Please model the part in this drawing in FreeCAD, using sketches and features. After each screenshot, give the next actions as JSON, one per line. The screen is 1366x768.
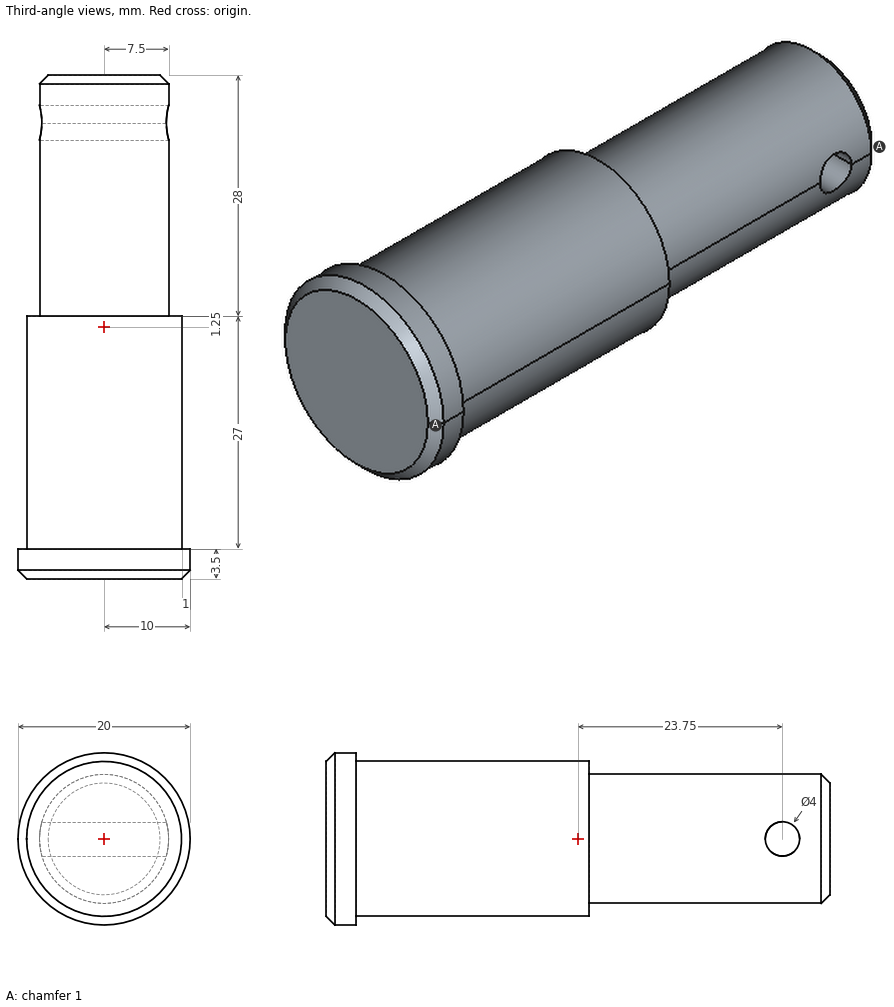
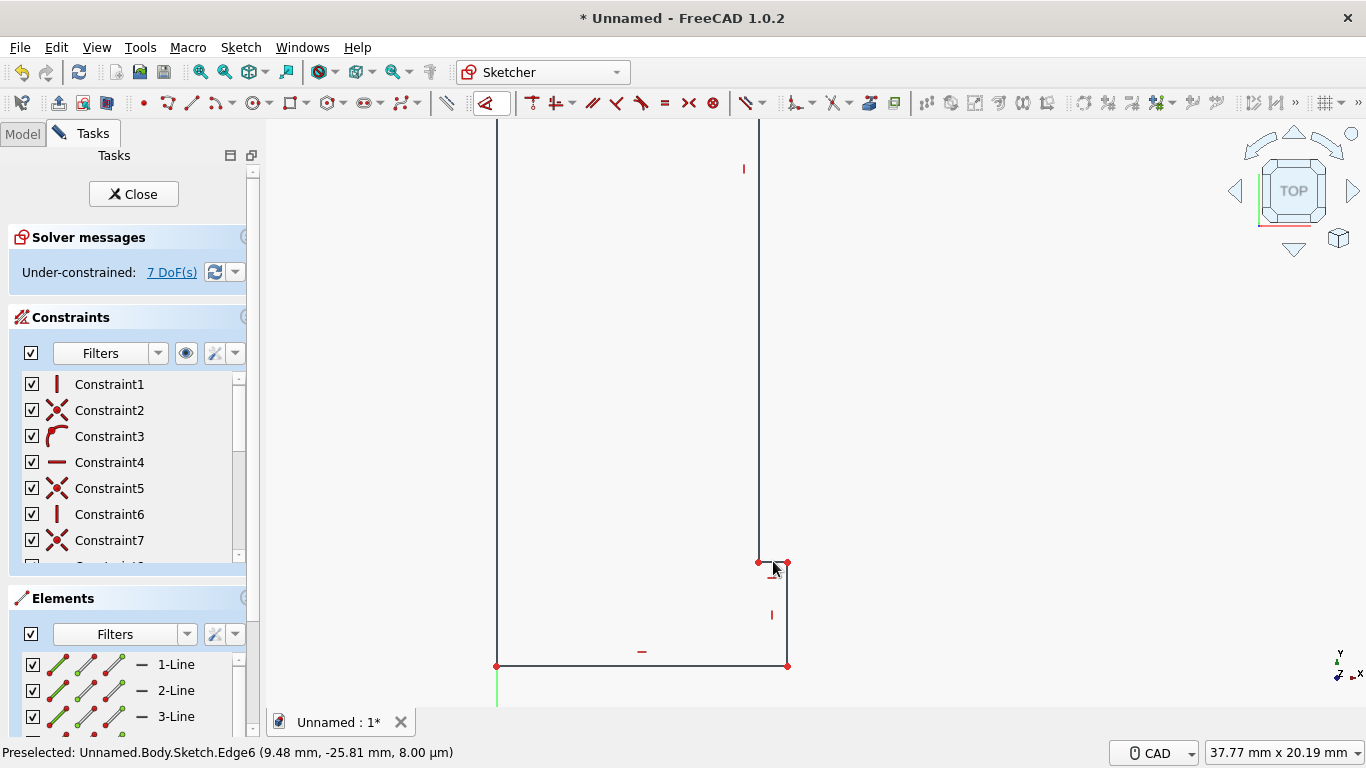
{"action": "left_click", "coordinate": [486, 104]}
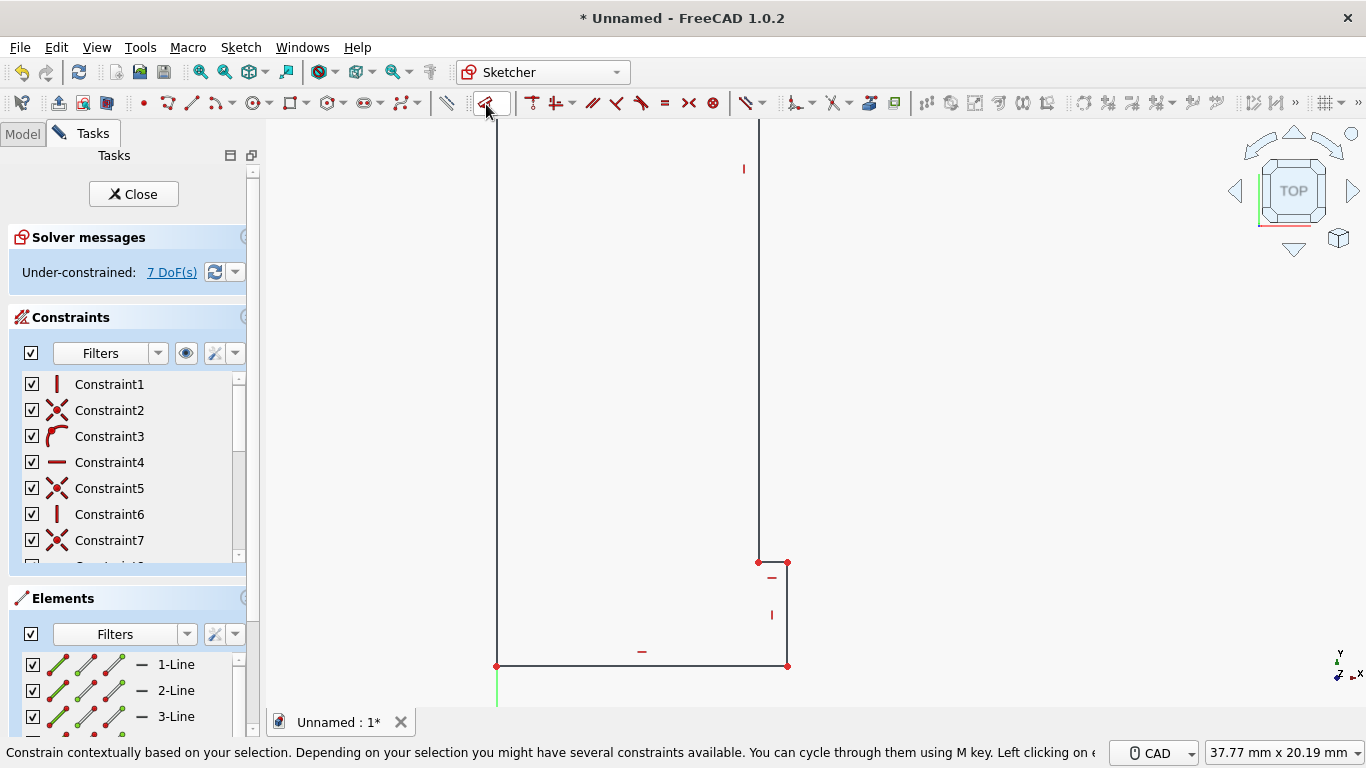
{"action": "scroll", "coordinate": [776, 562], "scroll_direction": "up", "scroll_amount": 2}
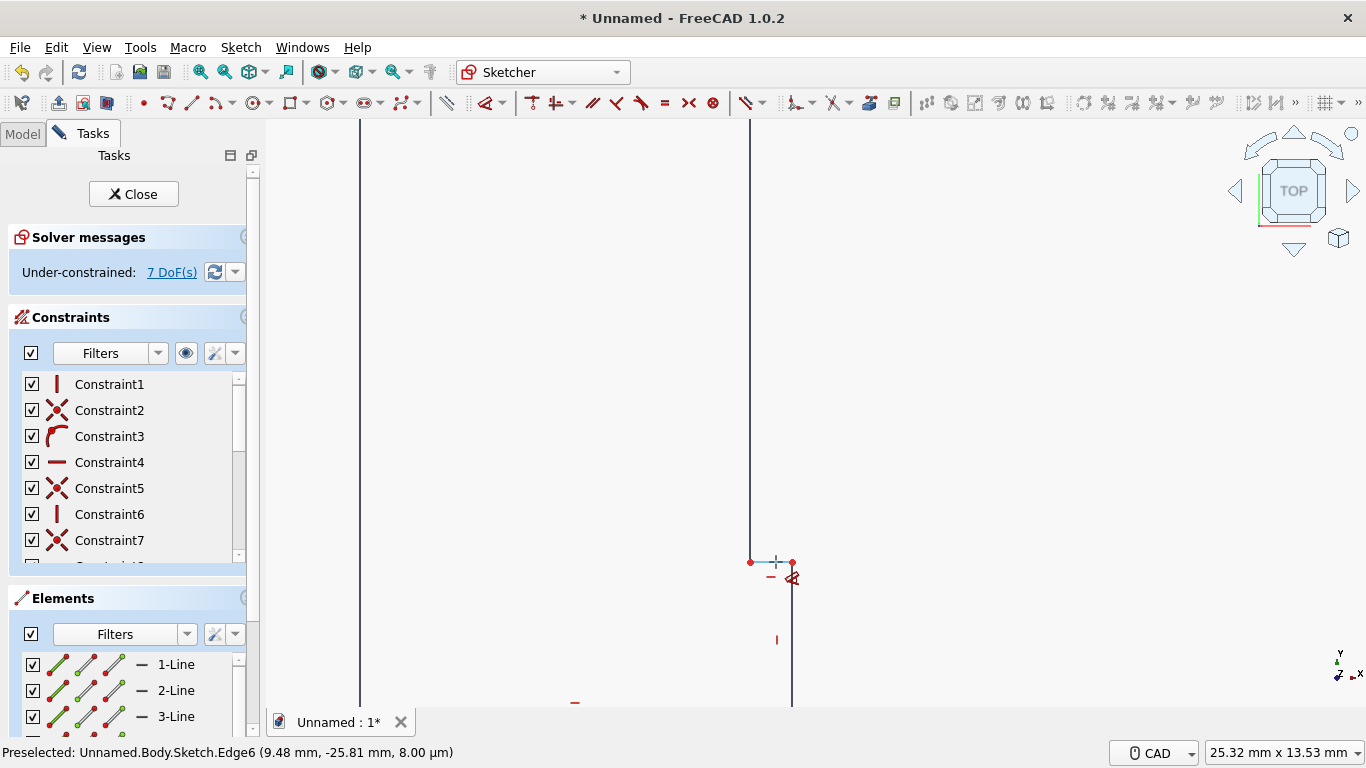
{"action": "left_click", "coordinate": [775, 562]}
{"action": "left_click", "coordinate": [771, 596]}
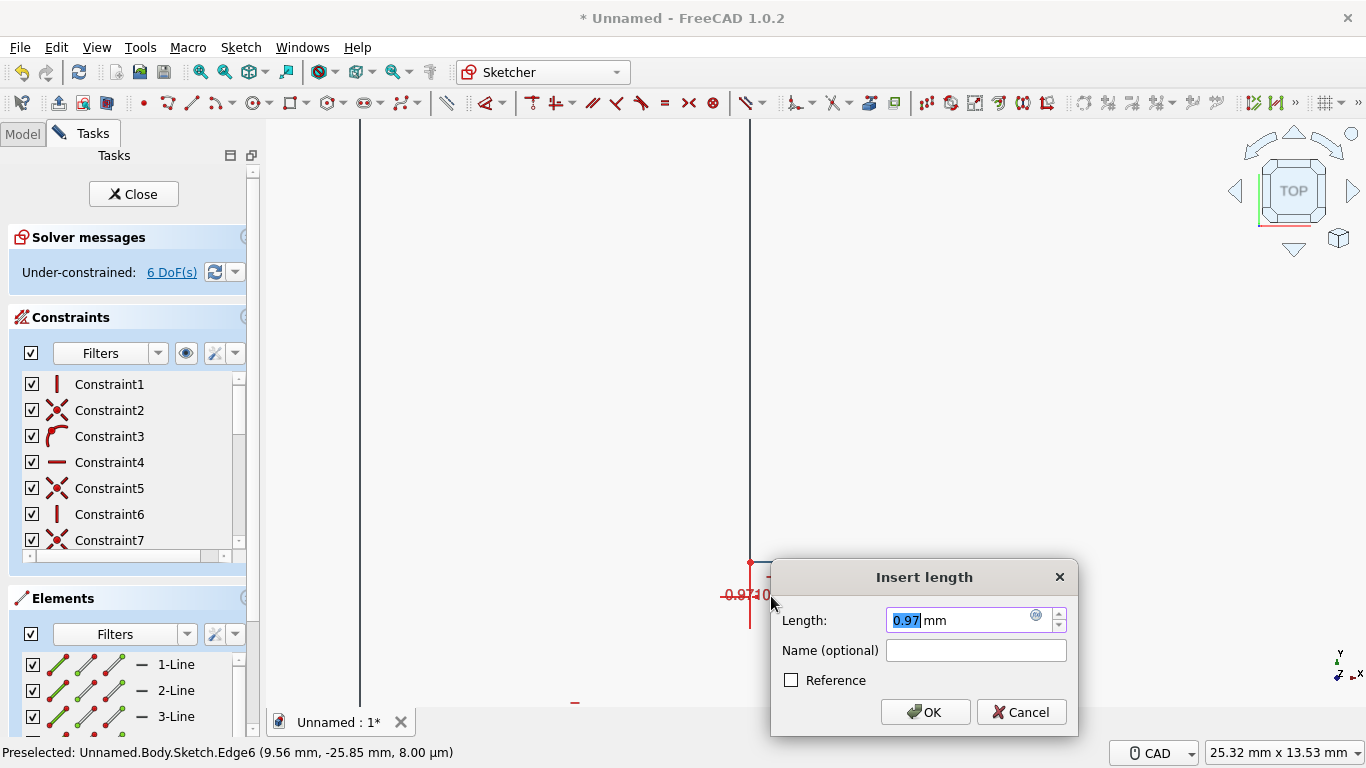
{"action": "type", "text": "1"}
{"action": "key", "text": "Return"}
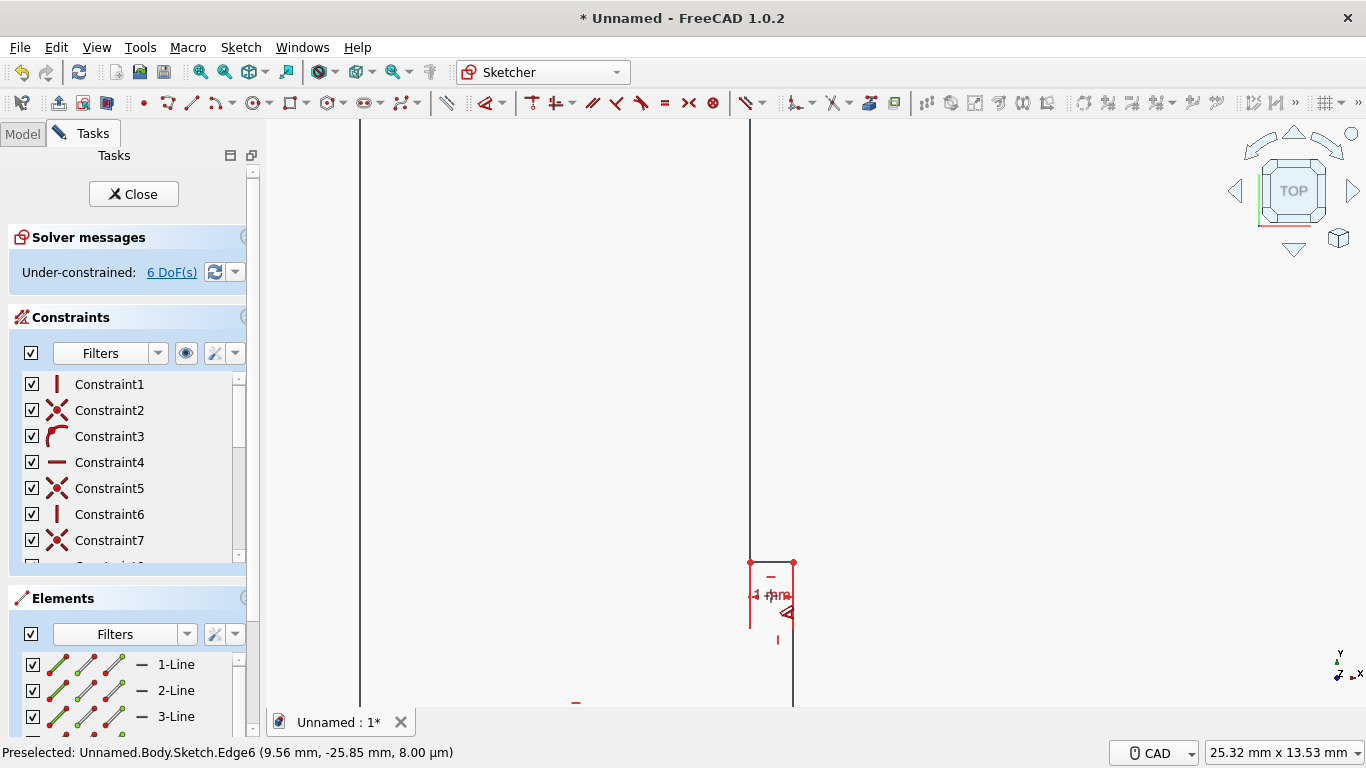
{"action": "scroll", "coordinate": [774, 565], "scroll_direction": "down", "scroll_amount": 10}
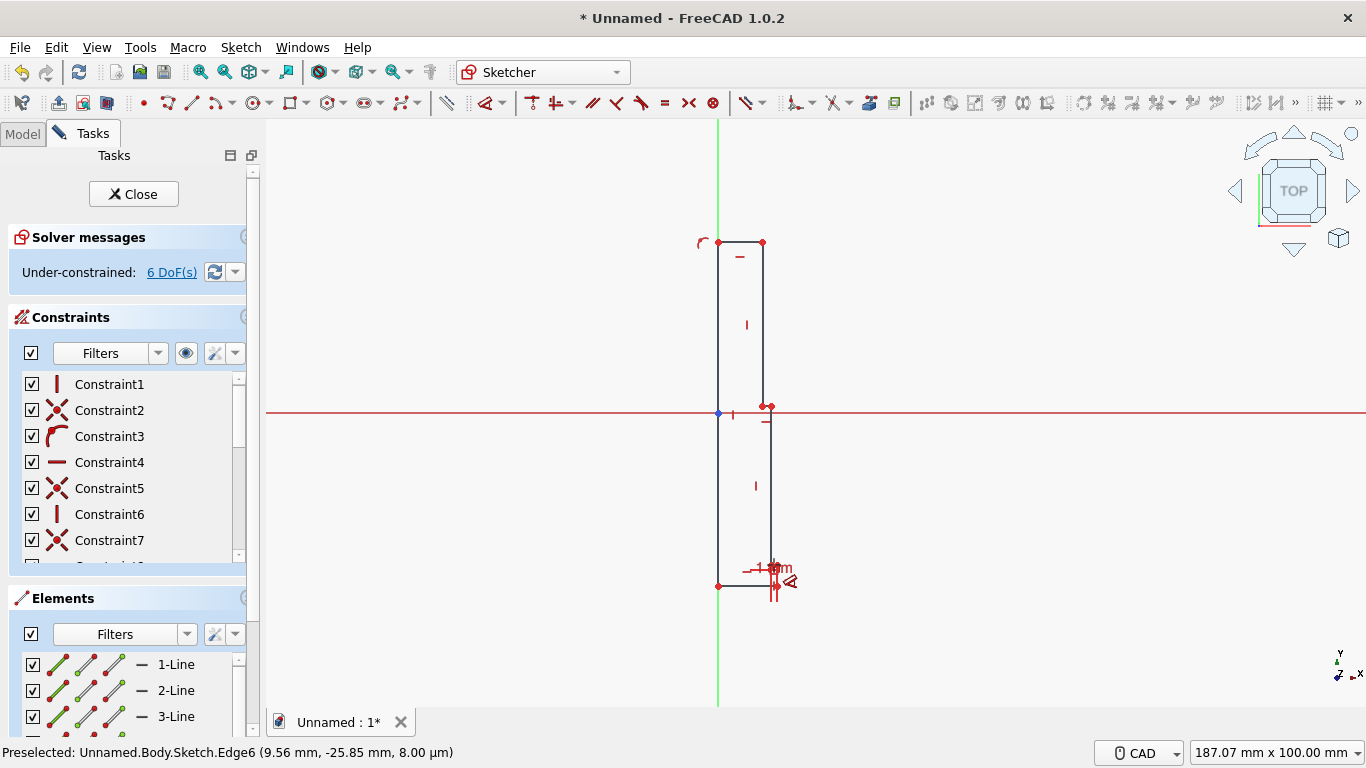
{"action": "left_click", "coordinate": [763, 357]}
{"action": "left_click", "coordinate": [797, 324]}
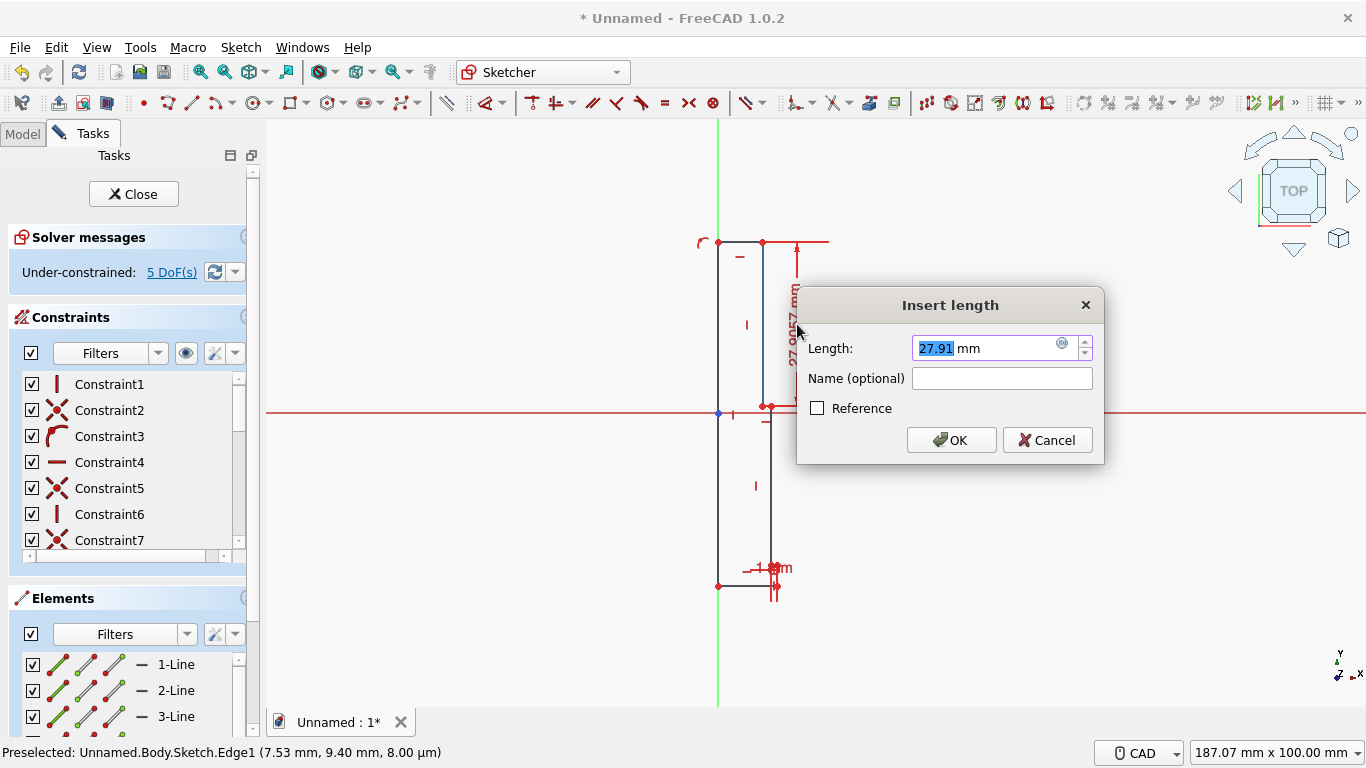
{"action": "type", "text": "28"}
{"action": "key", "text": "Return"}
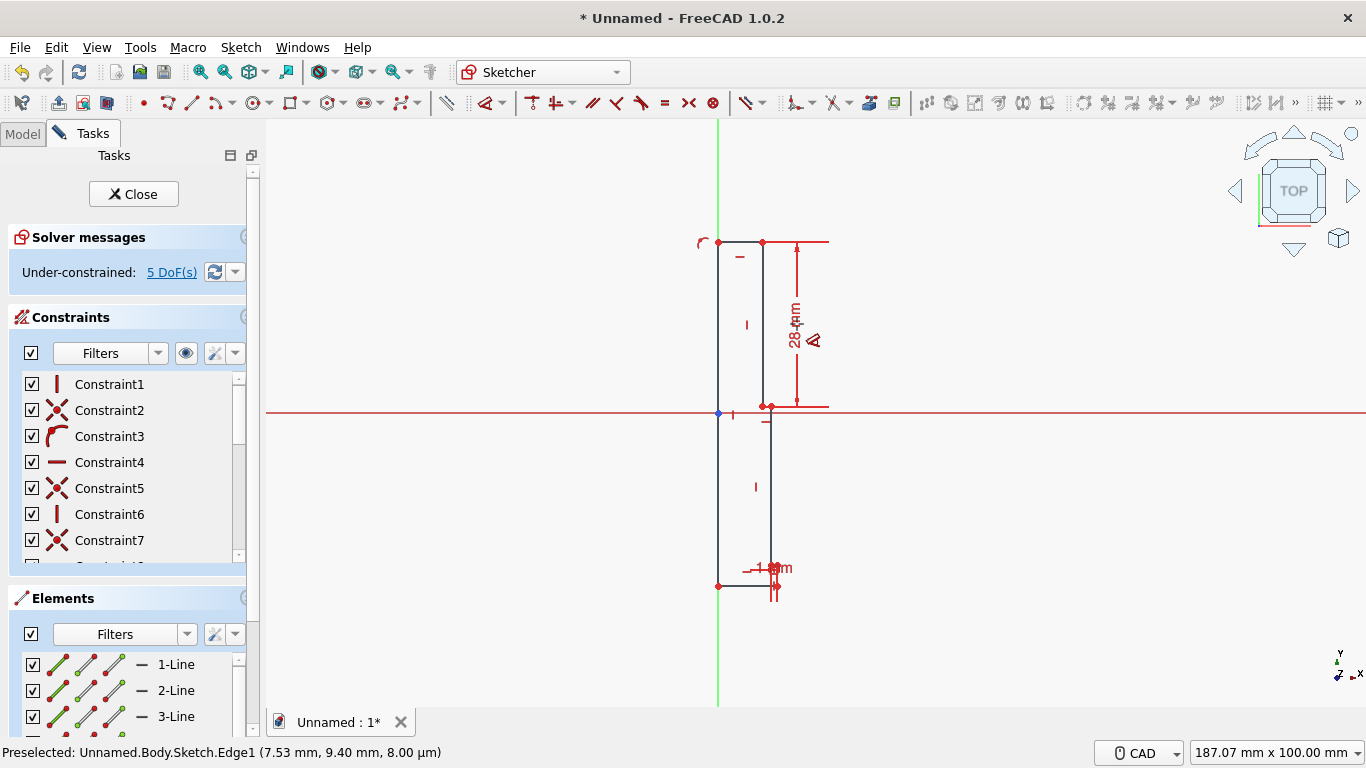
{"action": "left_click", "coordinate": [736, 586]}
{"action": "left_click", "coordinate": [748, 620]}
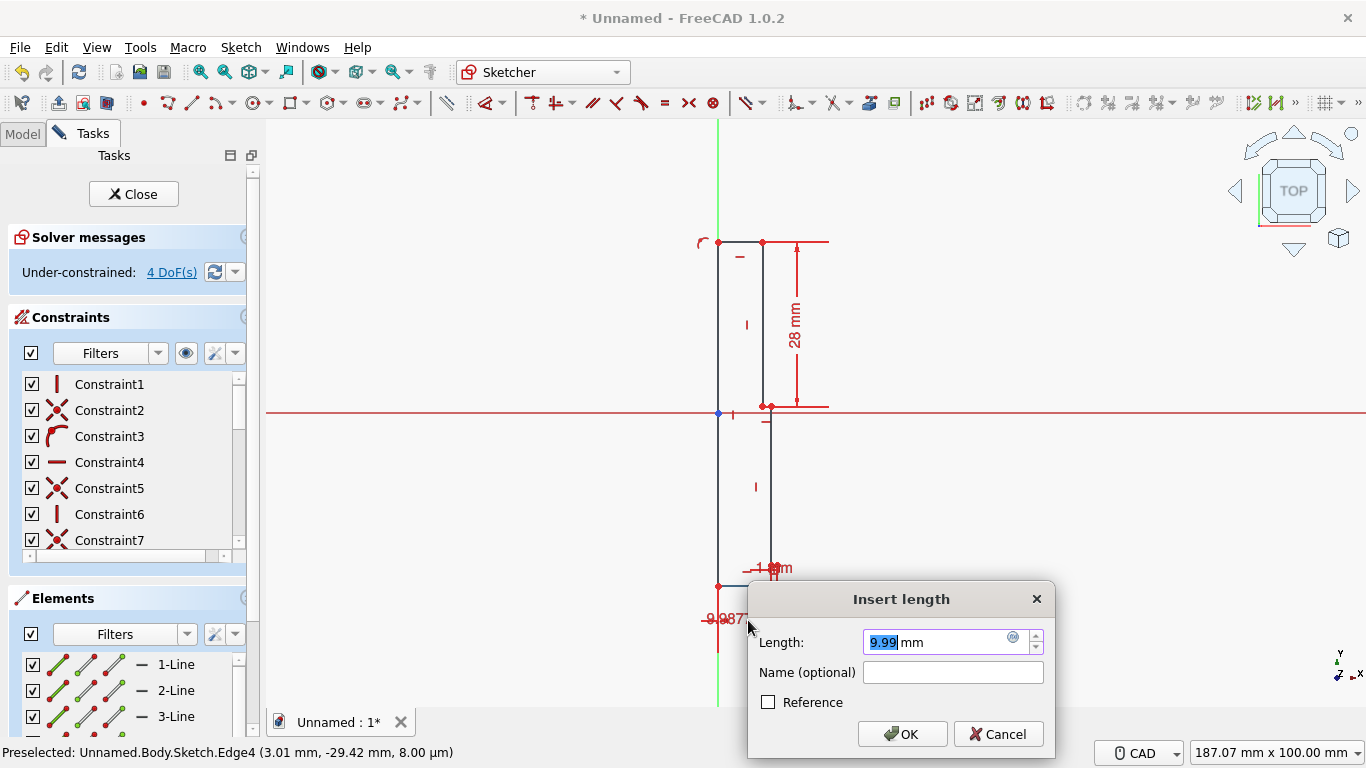
{"action": "type", "text": "10"}
{"action": "key", "text": "Return"}